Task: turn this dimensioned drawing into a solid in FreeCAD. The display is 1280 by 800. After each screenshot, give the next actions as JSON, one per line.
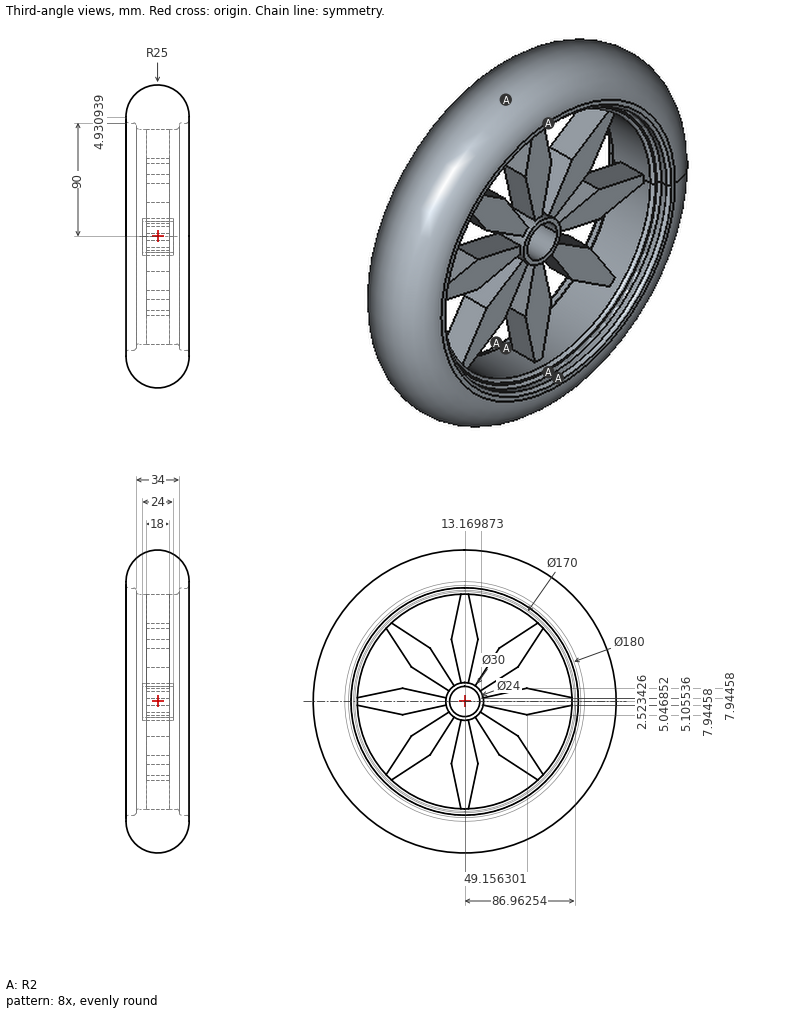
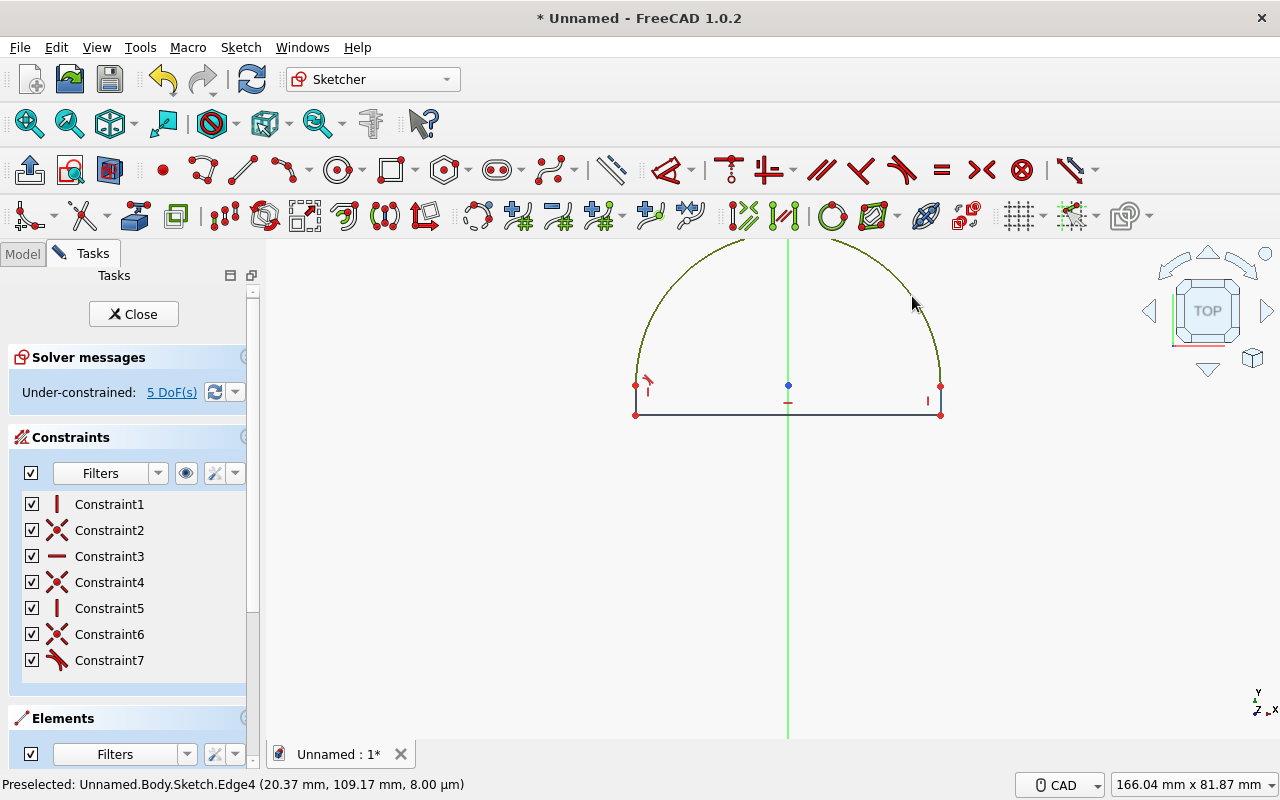
{"action": "left_click", "coordinate": [902, 170]}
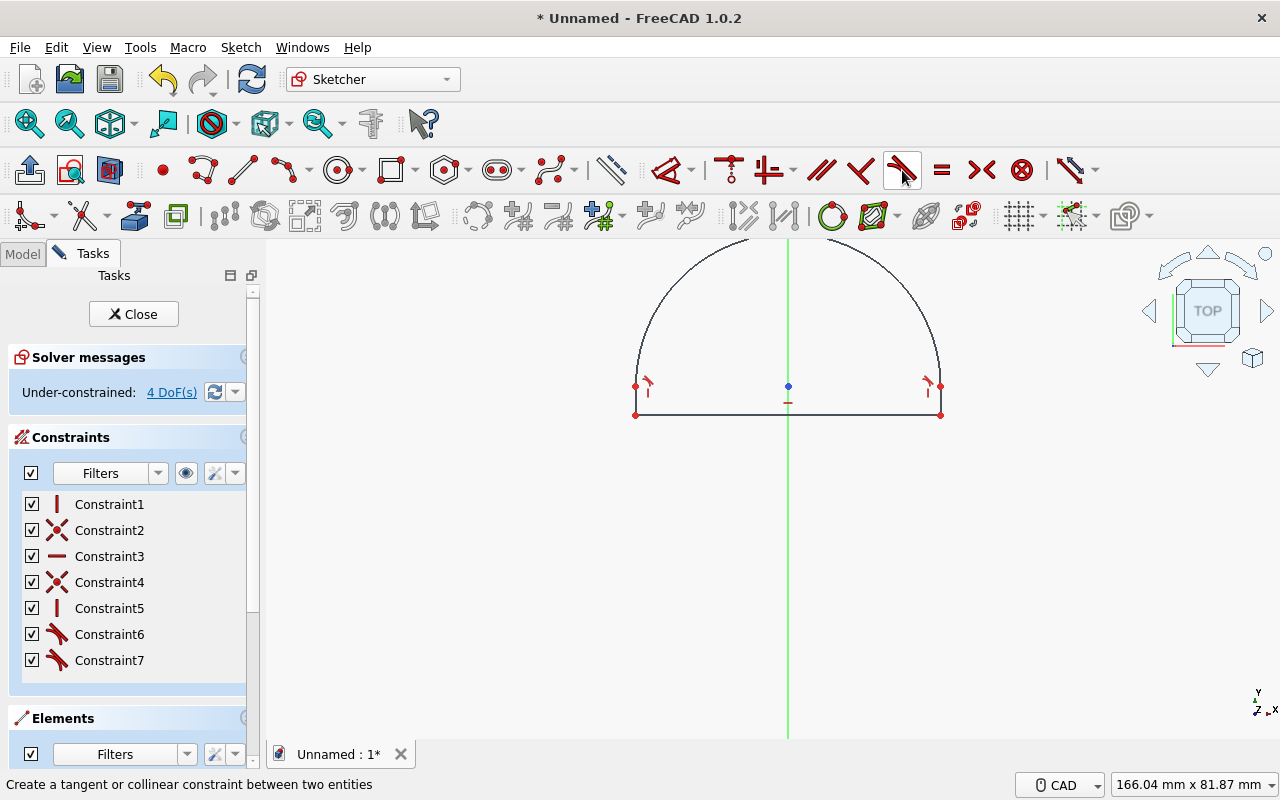
{"action": "left_click", "coordinate": [788, 386]}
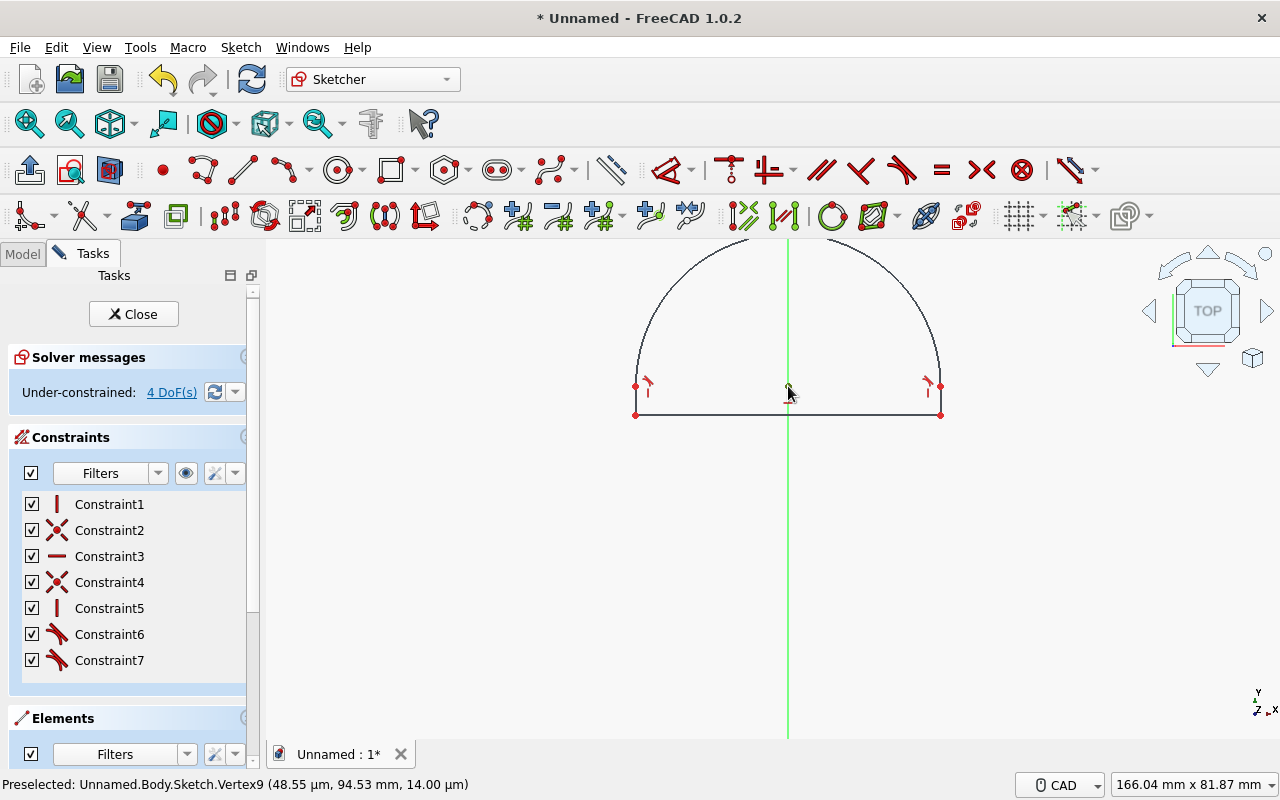
{"action": "left_click", "coordinate": [788, 679]}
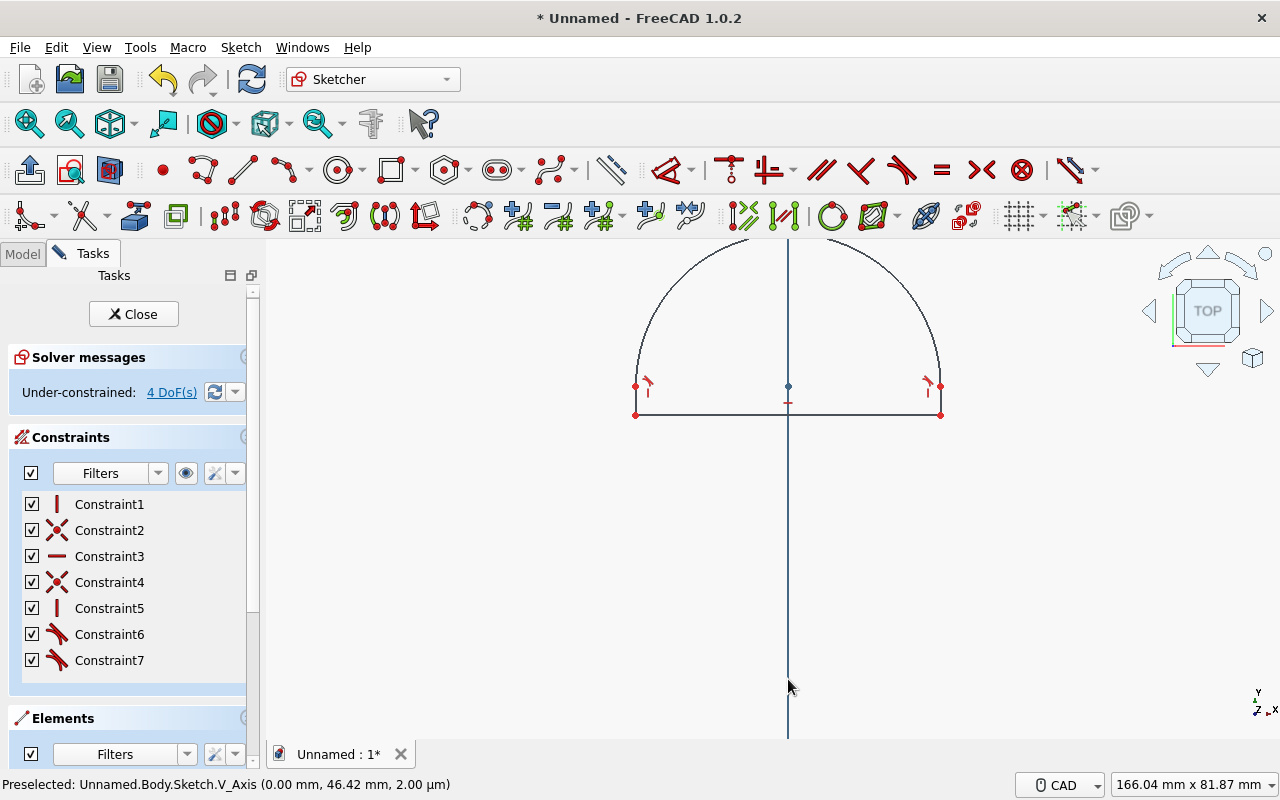
{"action": "key", "text": "c"}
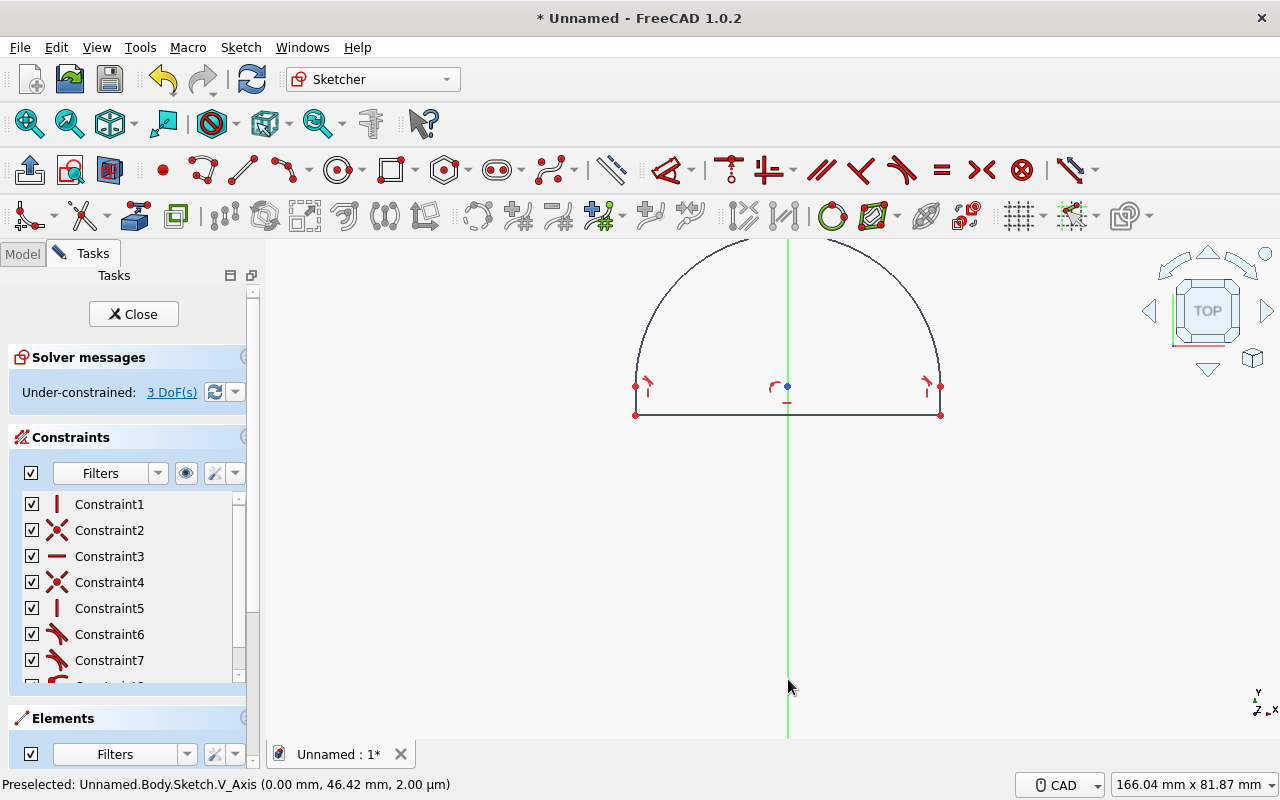
{"action": "left_click", "coordinate": [666, 170]}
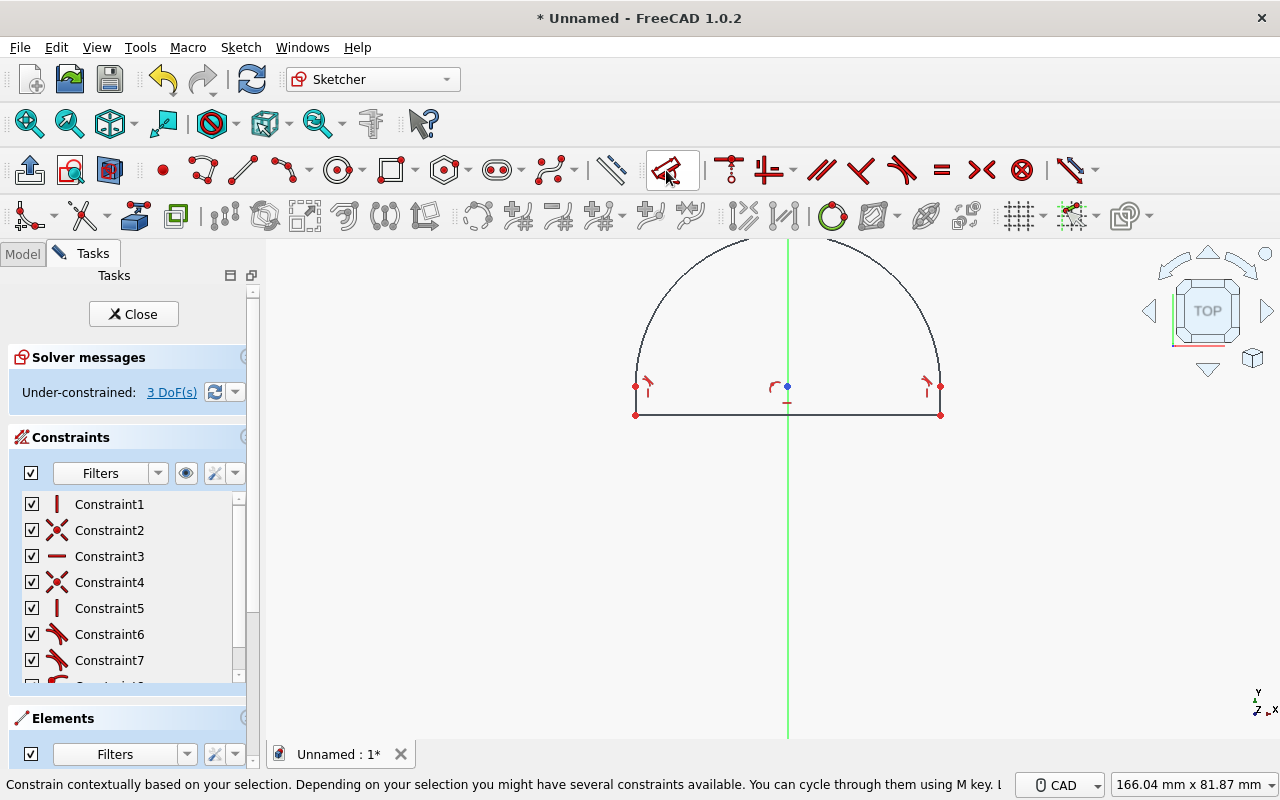
{"action": "left_click", "coordinate": [911, 297]}
{"action": "left_click", "coordinate": [937, 278]}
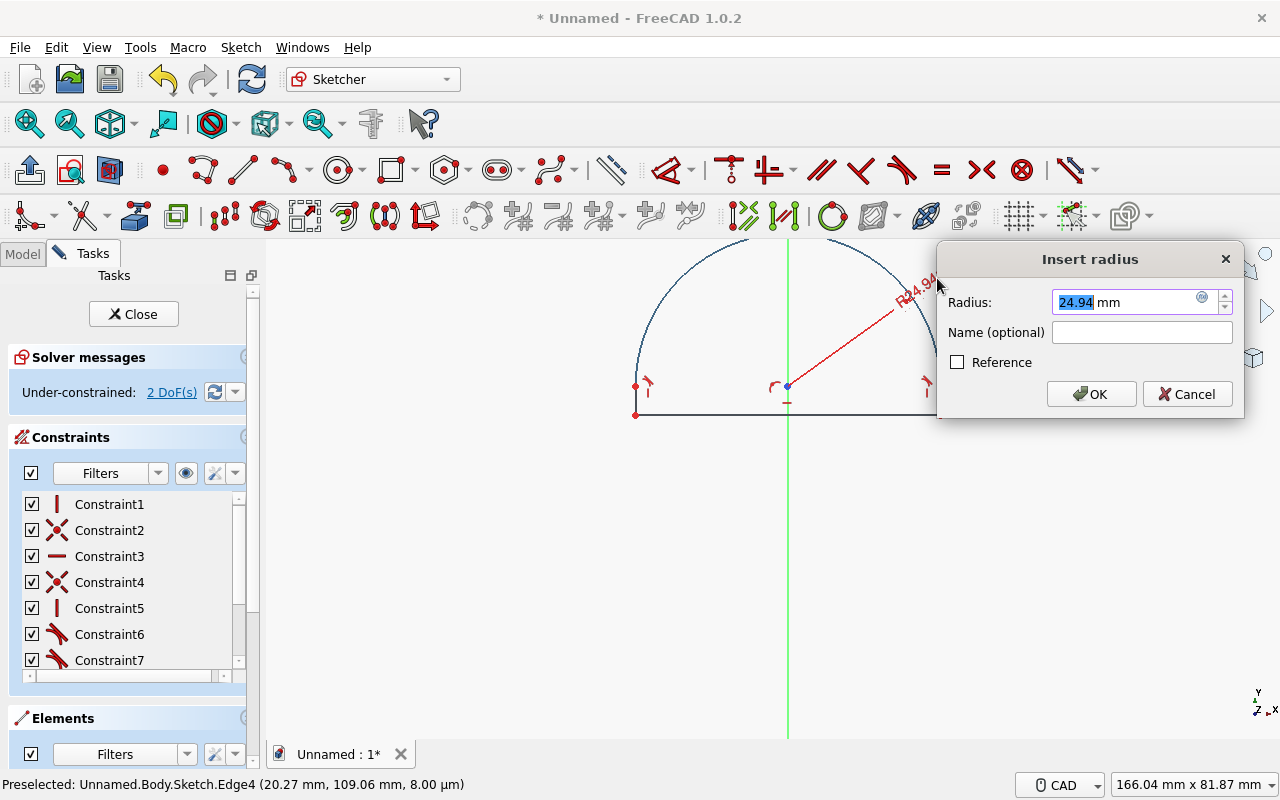
{"action": "type", "text": "25"}
{"action": "key", "text": "Return"}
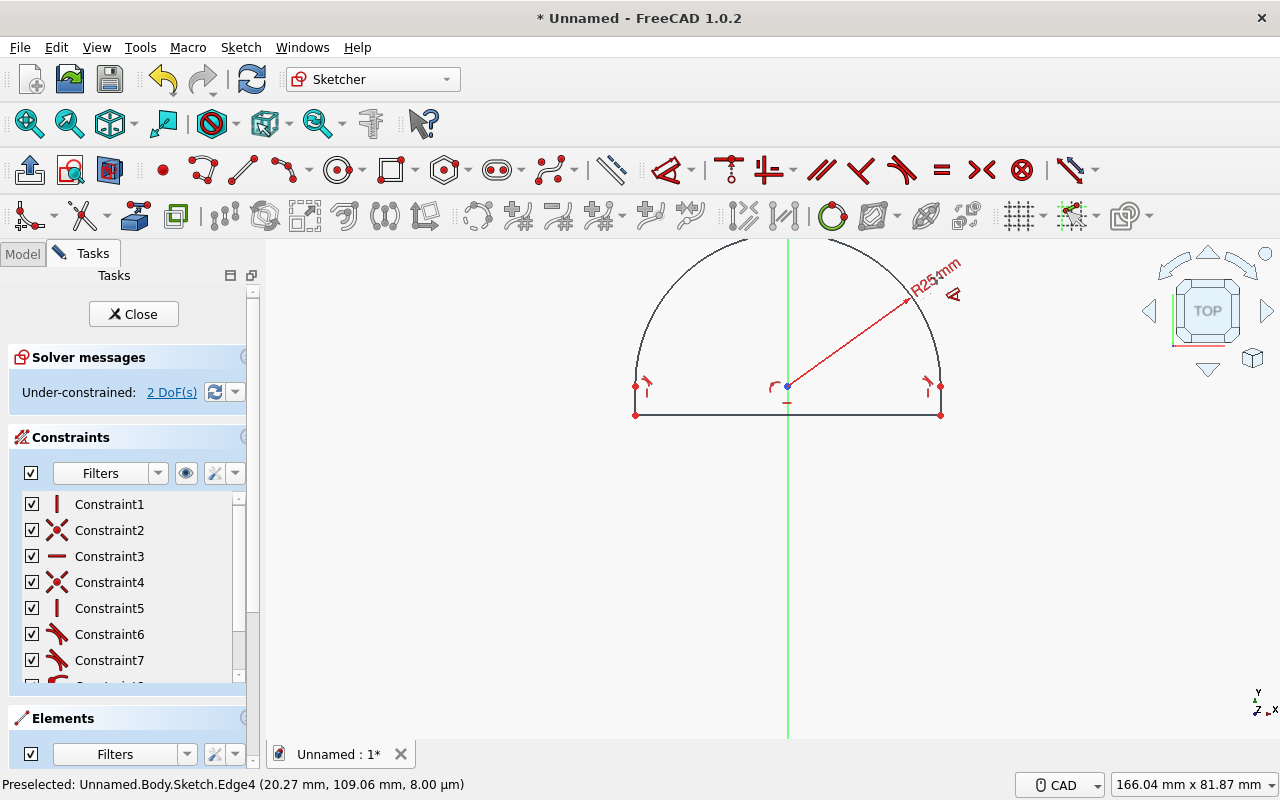
{"action": "left_click", "coordinate": [635, 415]}
{"action": "left_click", "coordinate": [601, 563]}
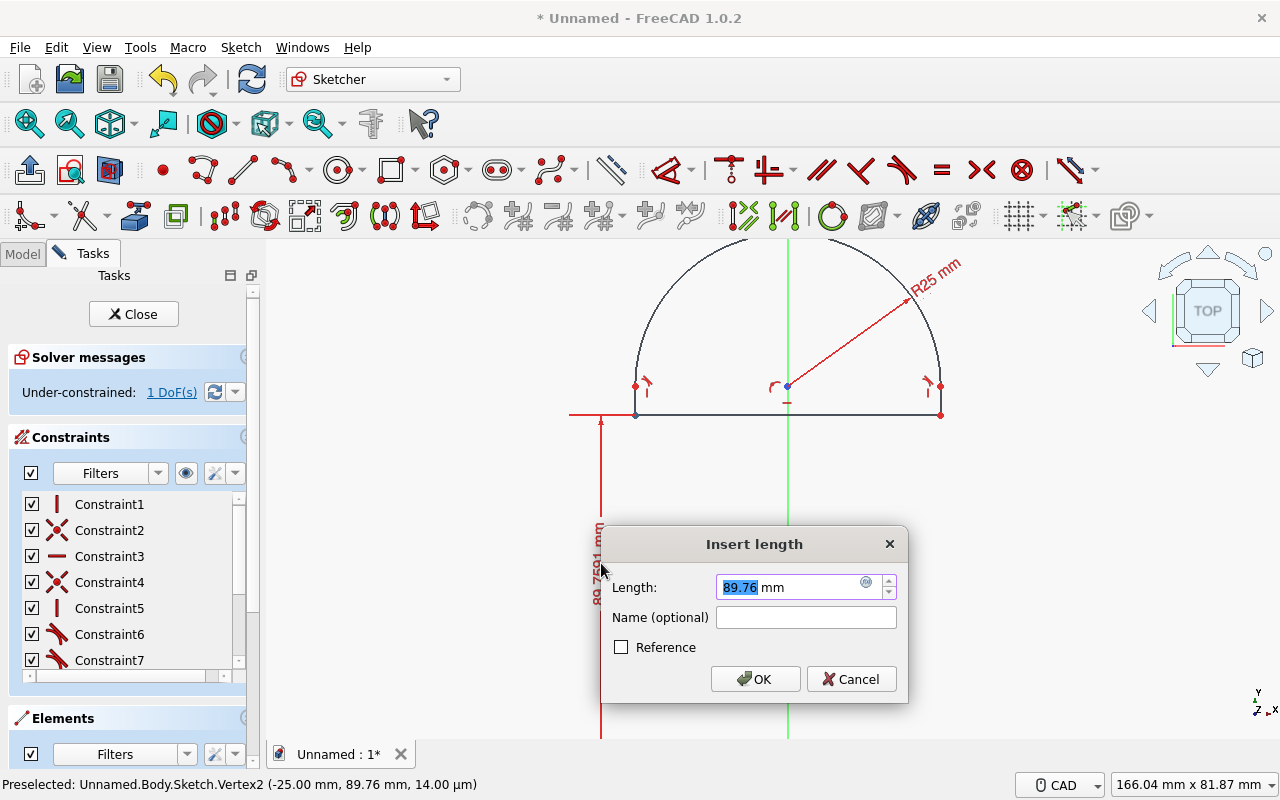
{"action": "type", "text": "90"}
{"action": "key", "text": "Return"}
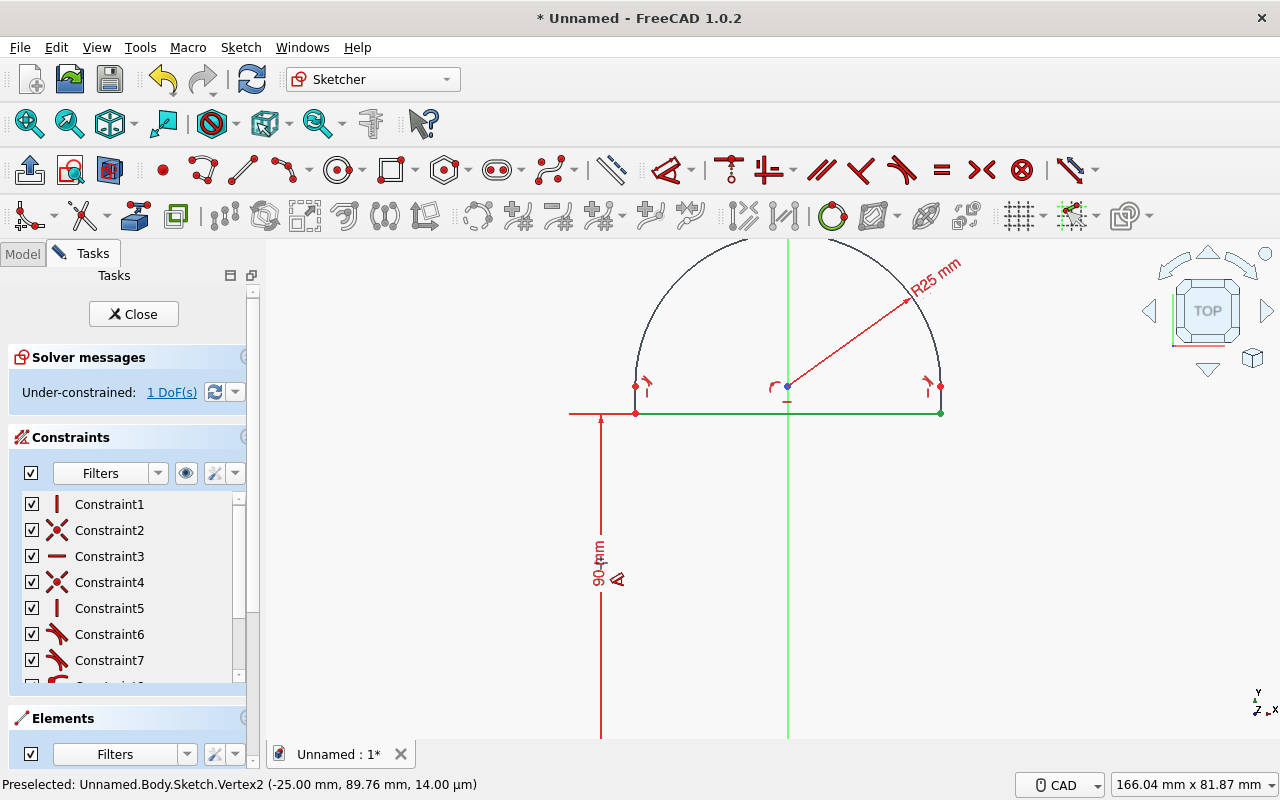
{"action": "scroll", "coordinate": [635, 397], "scroll_direction": "up", "scroll_amount": 2}